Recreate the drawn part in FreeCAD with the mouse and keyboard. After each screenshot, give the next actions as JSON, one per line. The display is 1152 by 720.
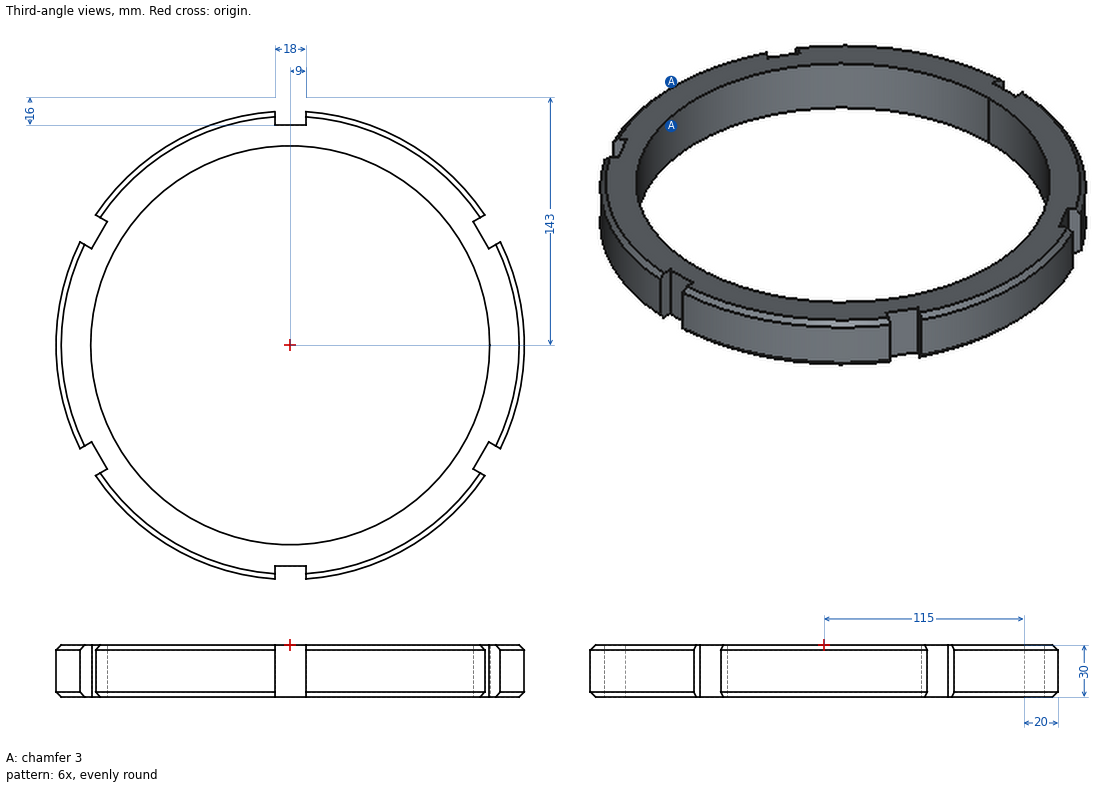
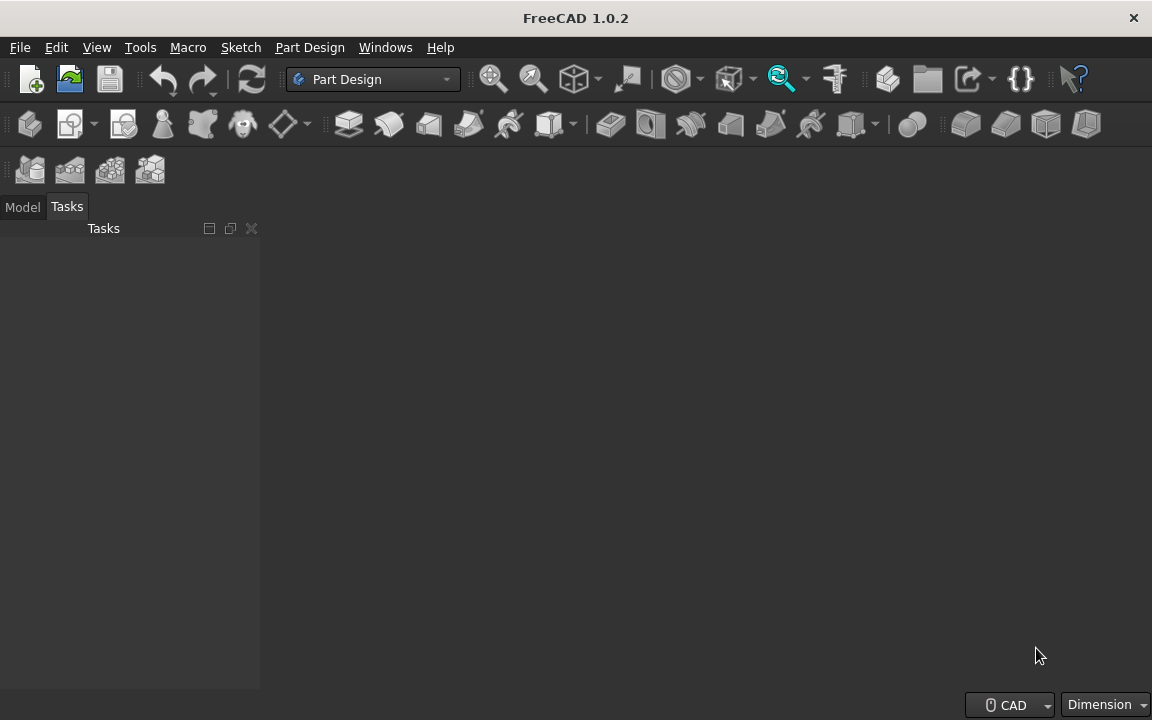
{"action": "left_click", "coordinate": [30, 80]}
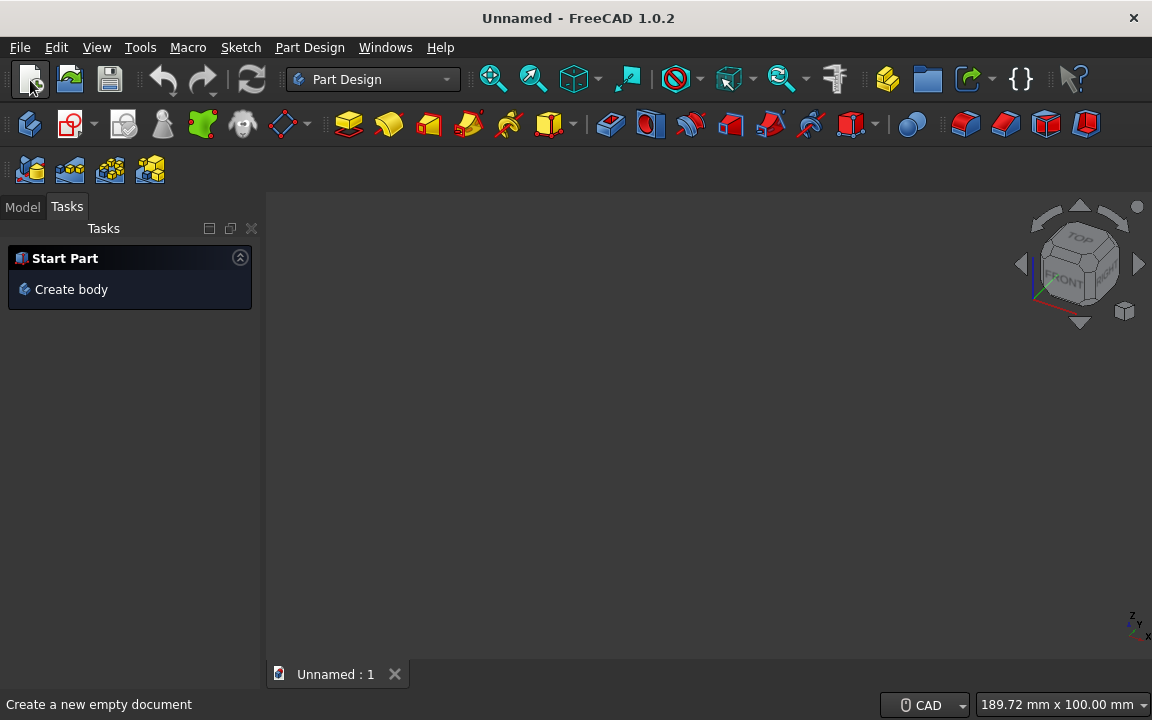
{"action": "left_click", "coordinate": [70, 124]}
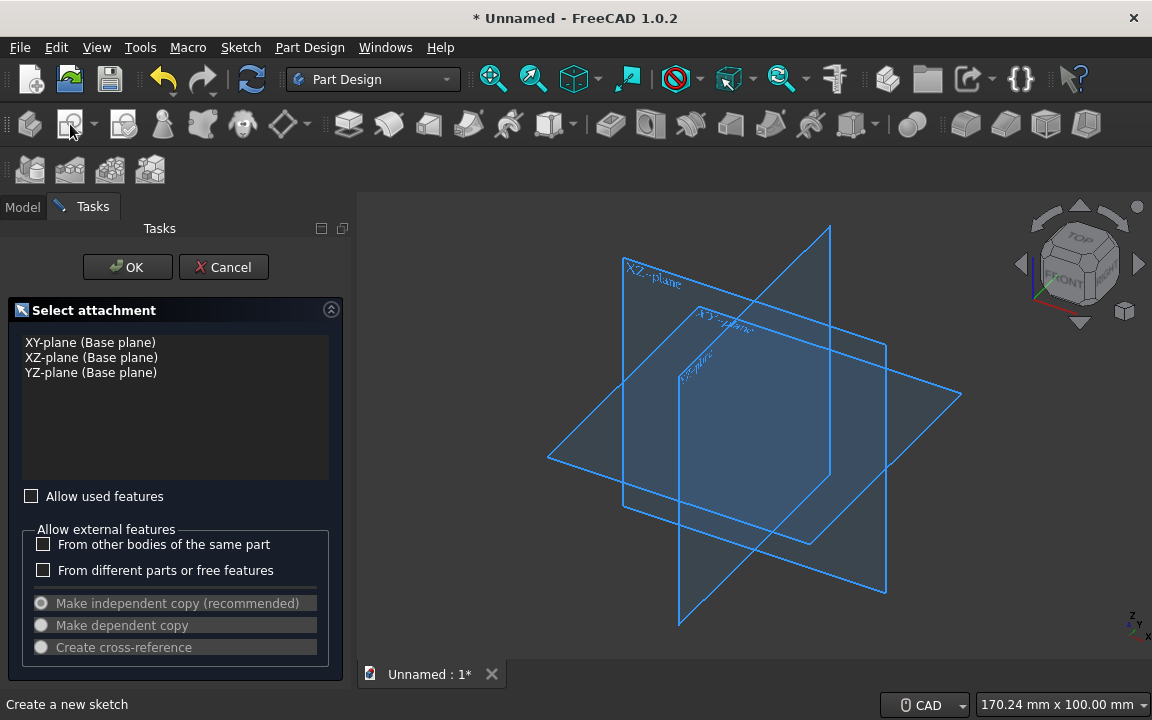
{"action": "left_click", "coordinate": [82, 372]}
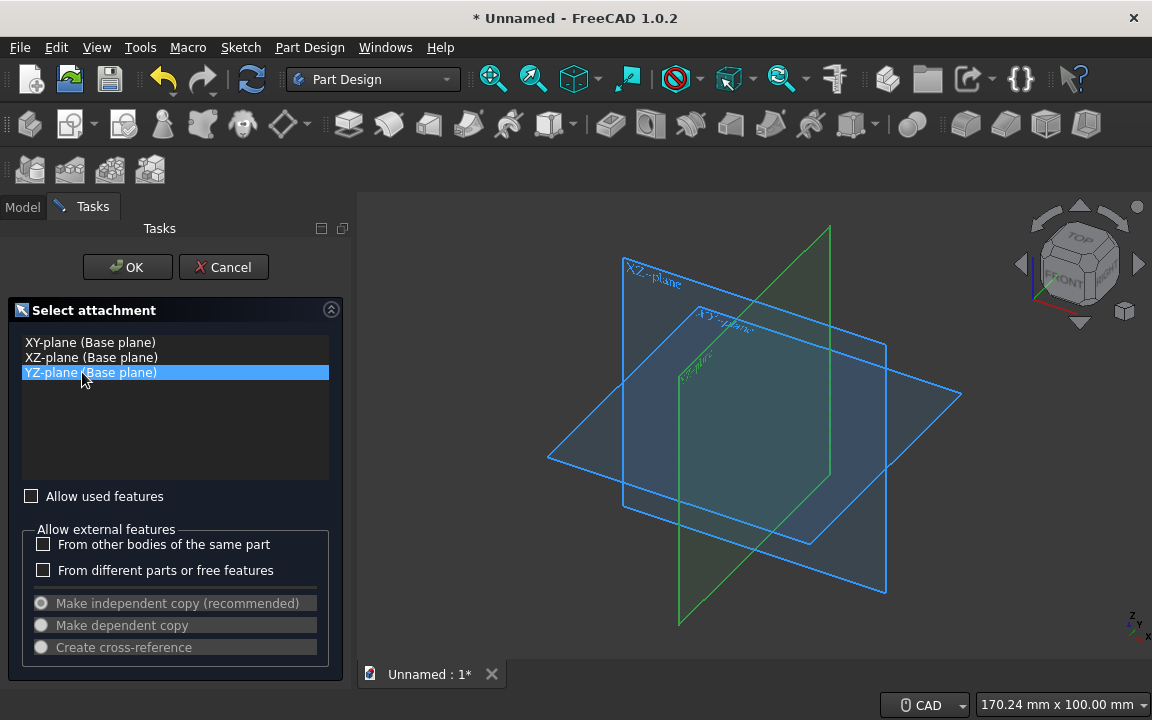
{"action": "left_click", "coordinate": [128, 267]}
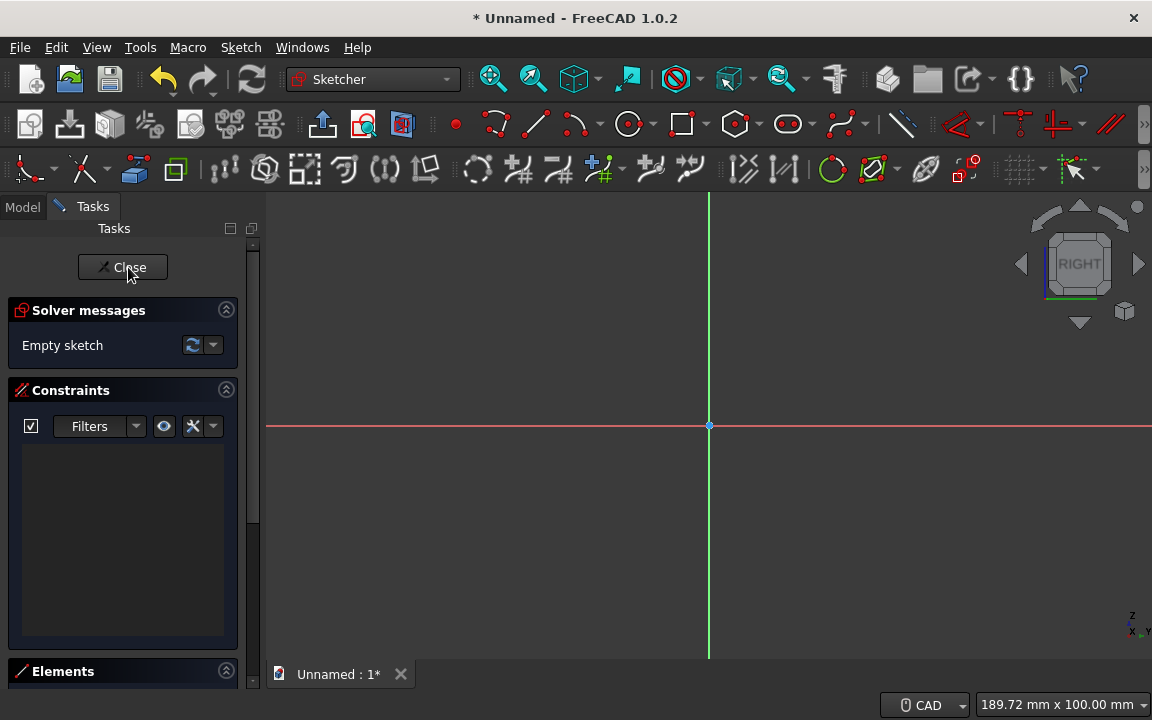
{"action": "scroll", "coordinate": [640, 426], "scroll_direction": "down", "scroll_amount": 5}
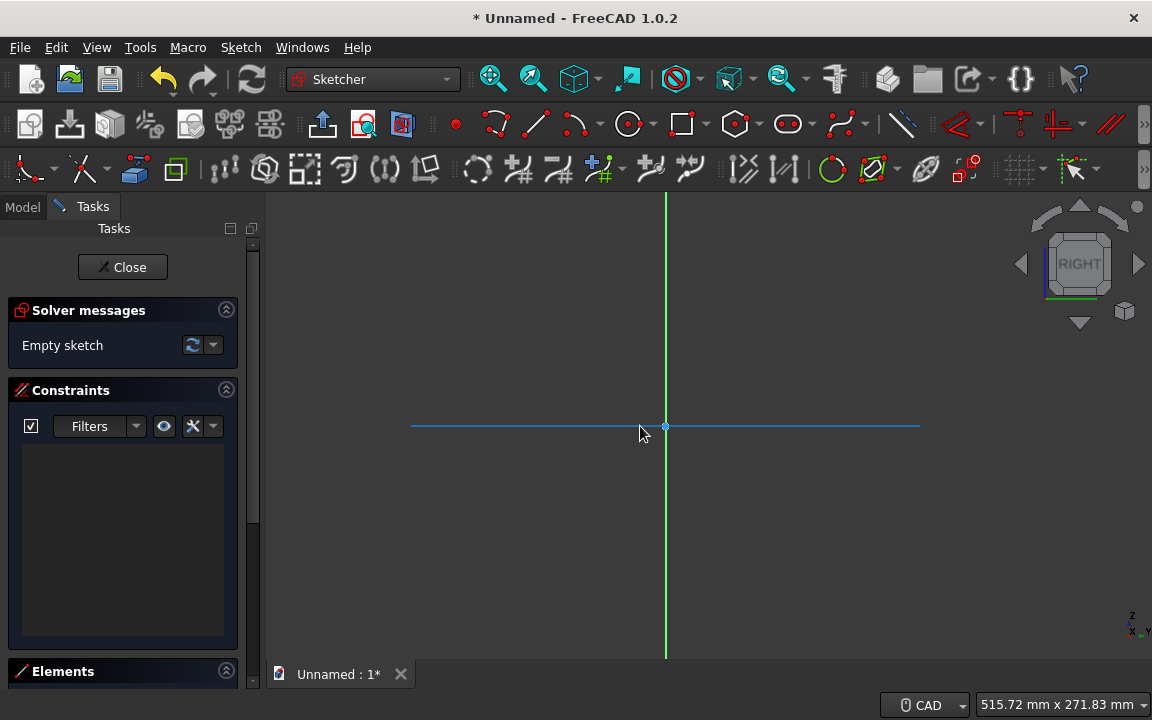
{"action": "scroll", "coordinate": [928, 457], "scroll_direction": "up", "scroll_amount": 9}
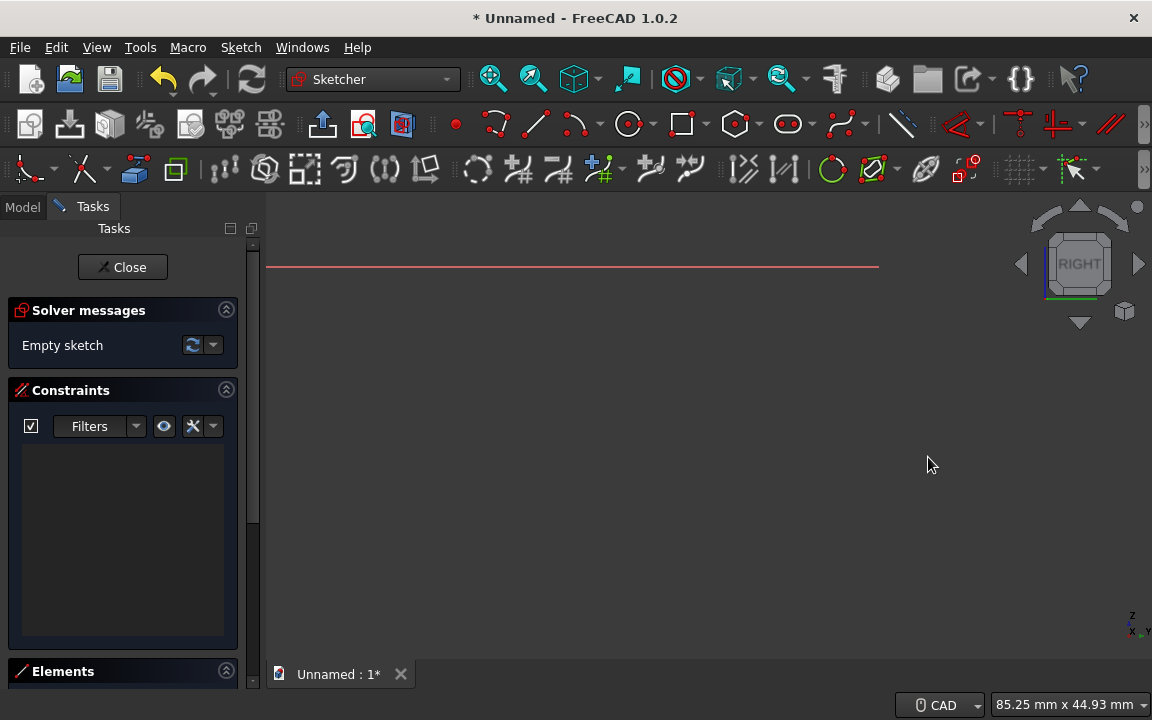
{"action": "left_click", "coordinate": [682, 124]}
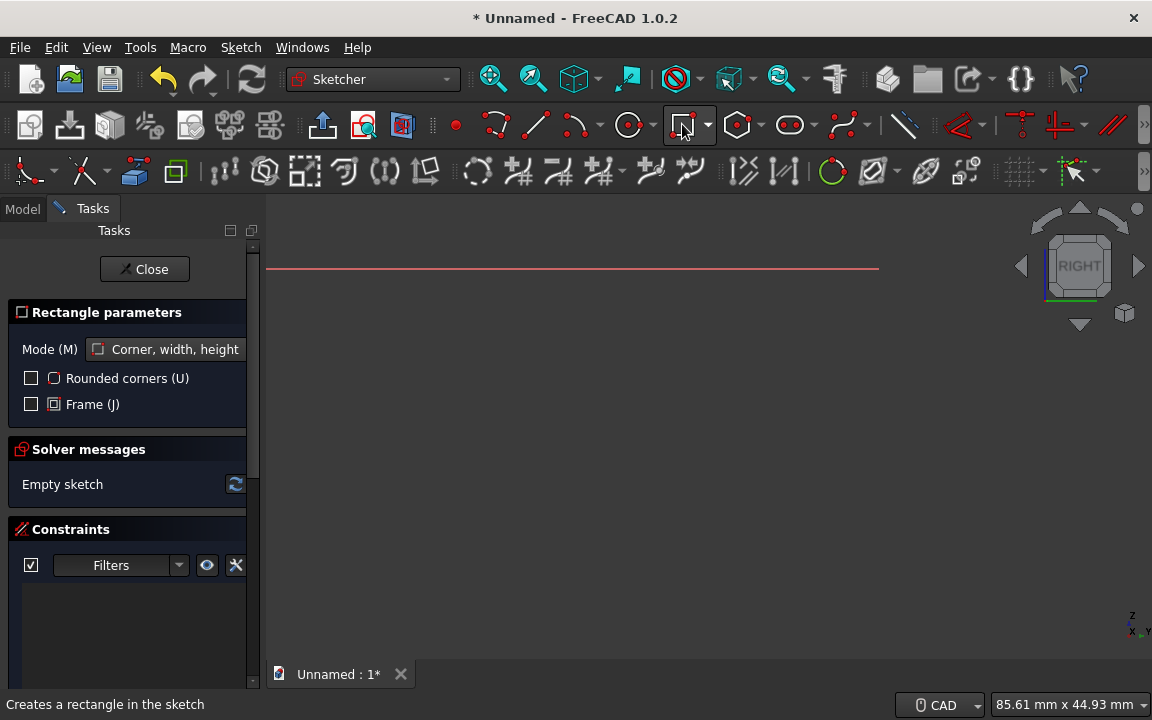
{"action": "left_click", "coordinate": [533, 269]}
{"action": "left_click", "coordinate": [740, 580]}
{"action": "key", "text": "Escape"}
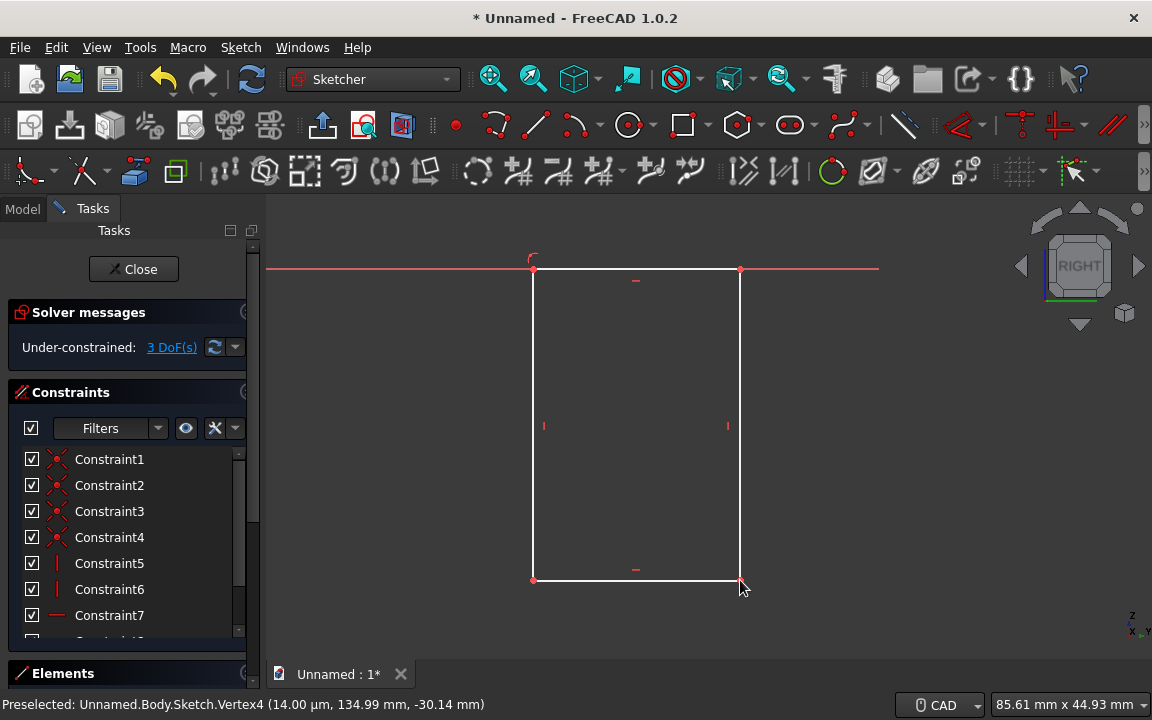
{"action": "left_click", "coordinate": [958, 126]}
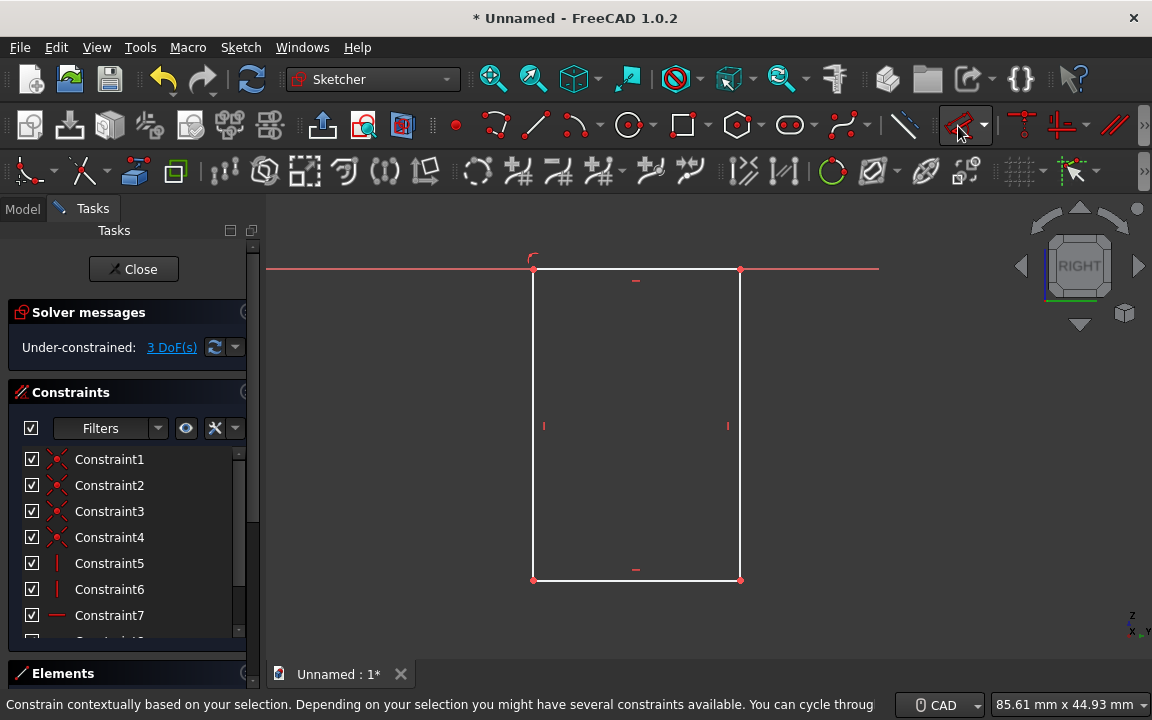
{"action": "left_click", "coordinate": [533, 363]}
{"action": "left_click", "coordinate": [499, 425]}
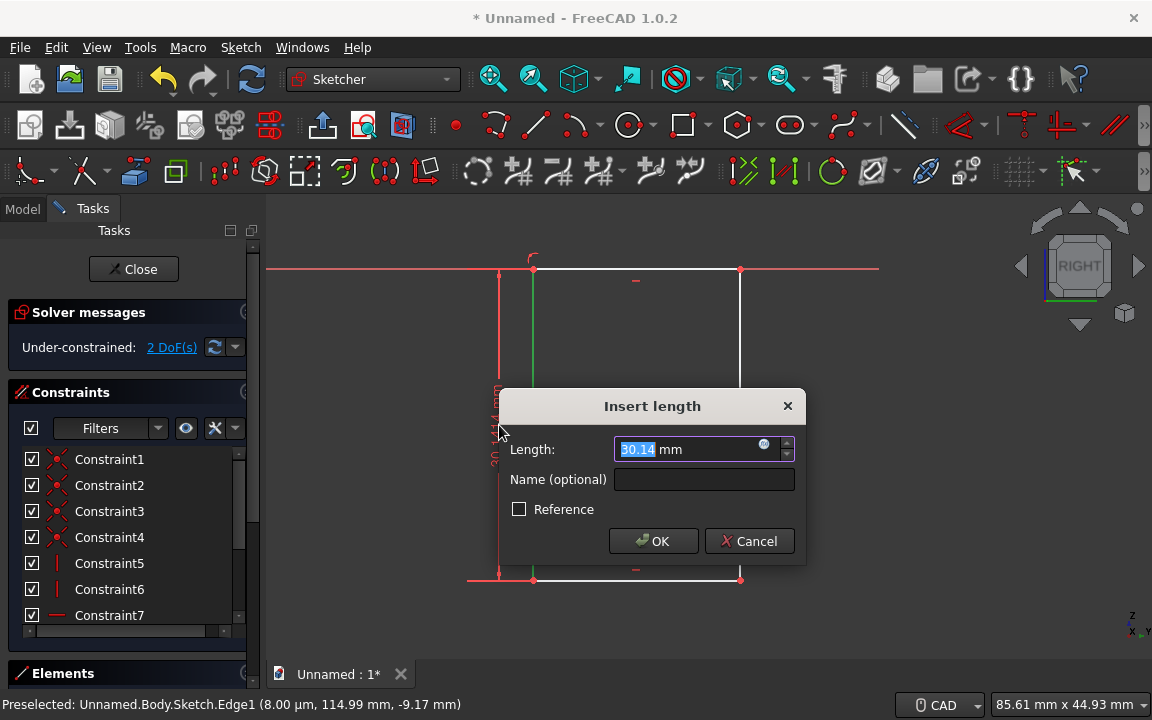
{"action": "type", "text": "30"}
{"action": "key", "text": "Return"}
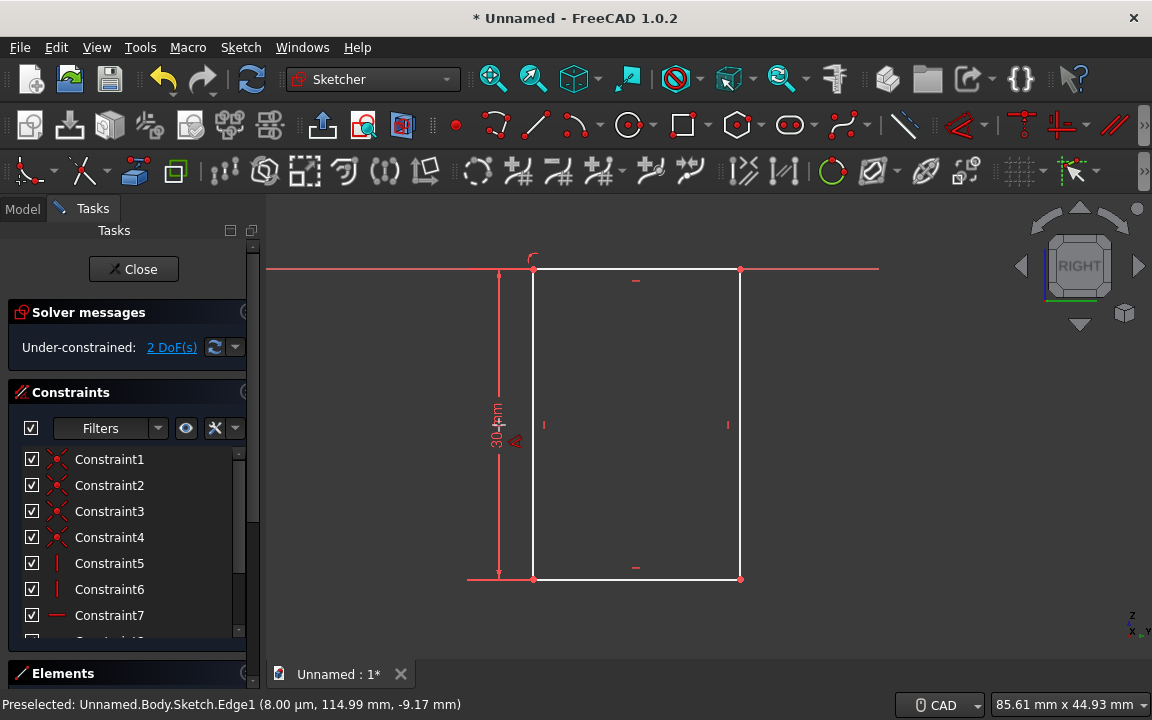
{"action": "left_click", "coordinate": [595, 580]}
{"action": "left_click", "coordinate": [637, 614]}